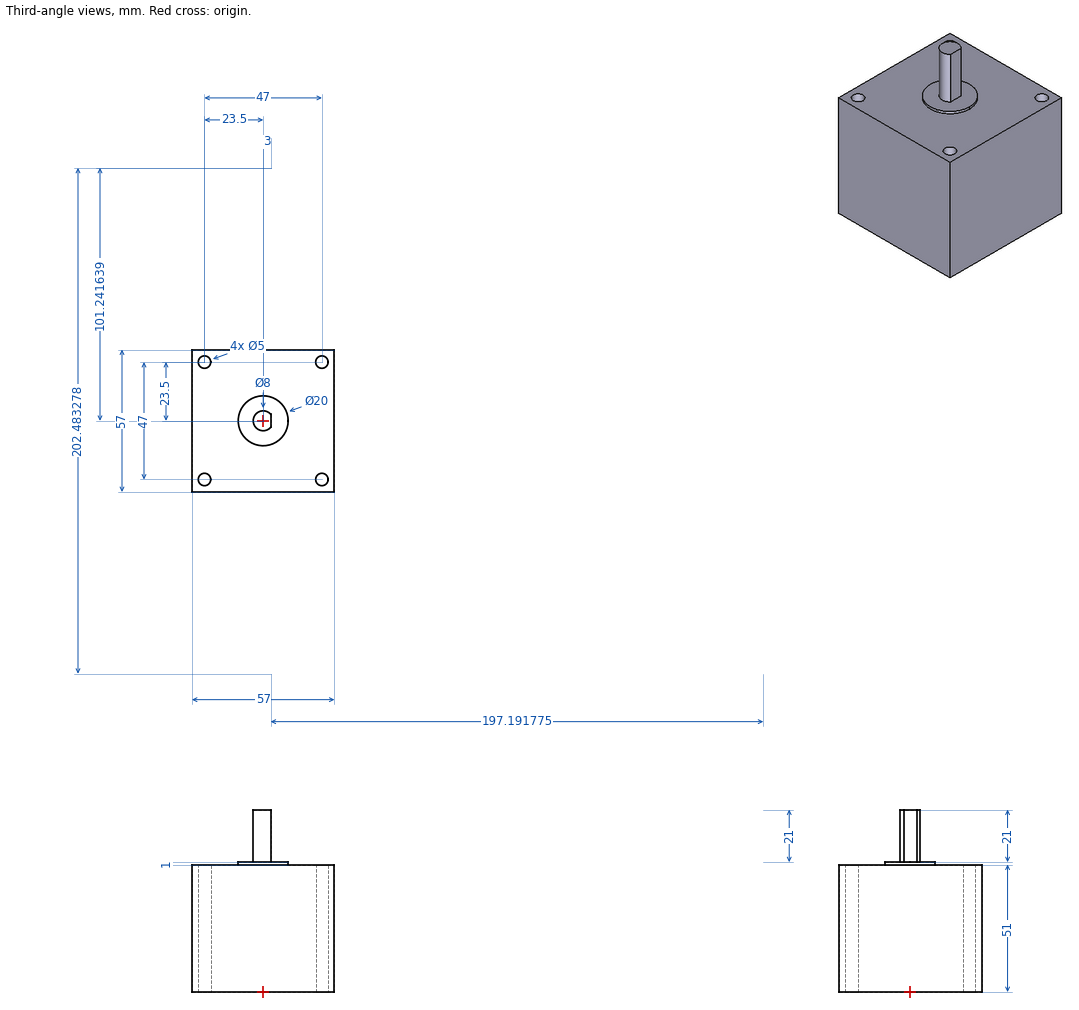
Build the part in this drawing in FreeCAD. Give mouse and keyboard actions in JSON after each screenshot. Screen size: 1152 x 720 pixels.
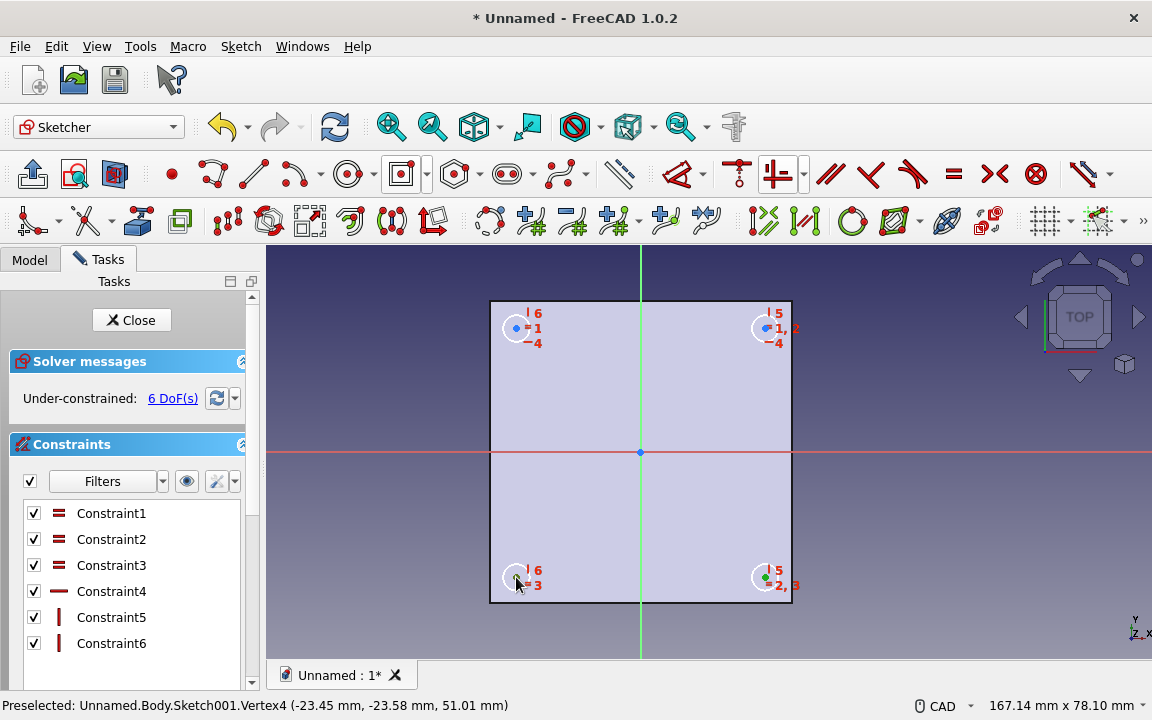
{"action": "left_click", "coordinate": [804, 174]}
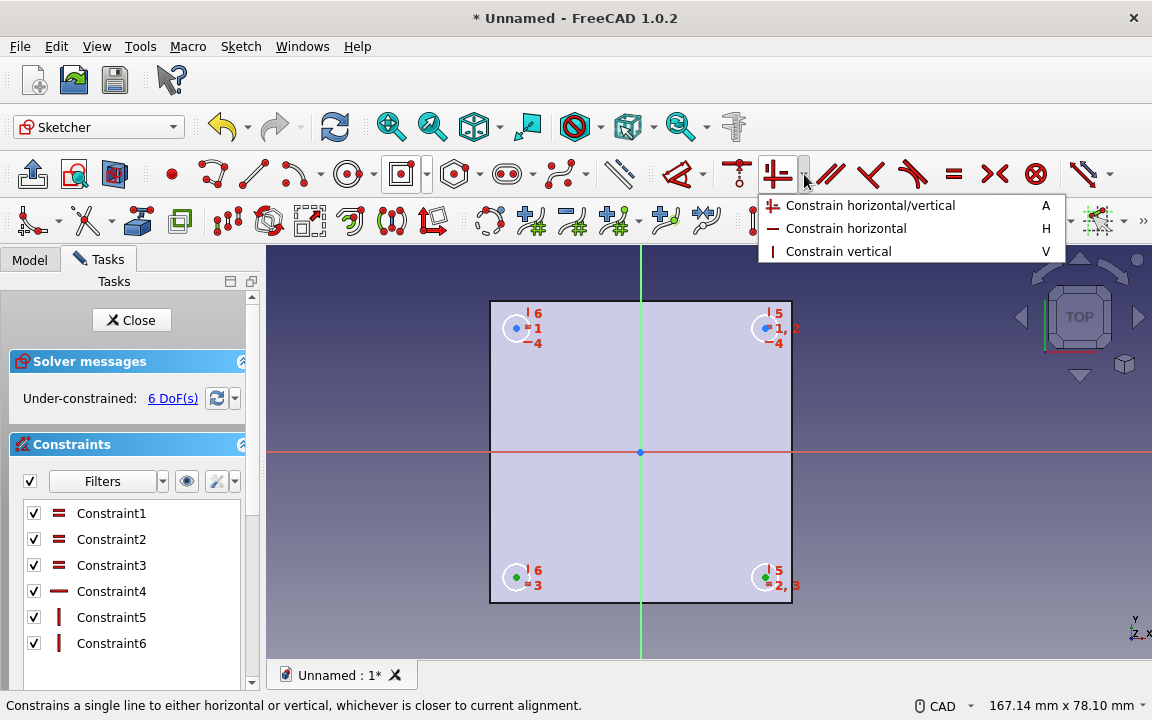
{"action": "left_click", "coordinate": [912, 228]}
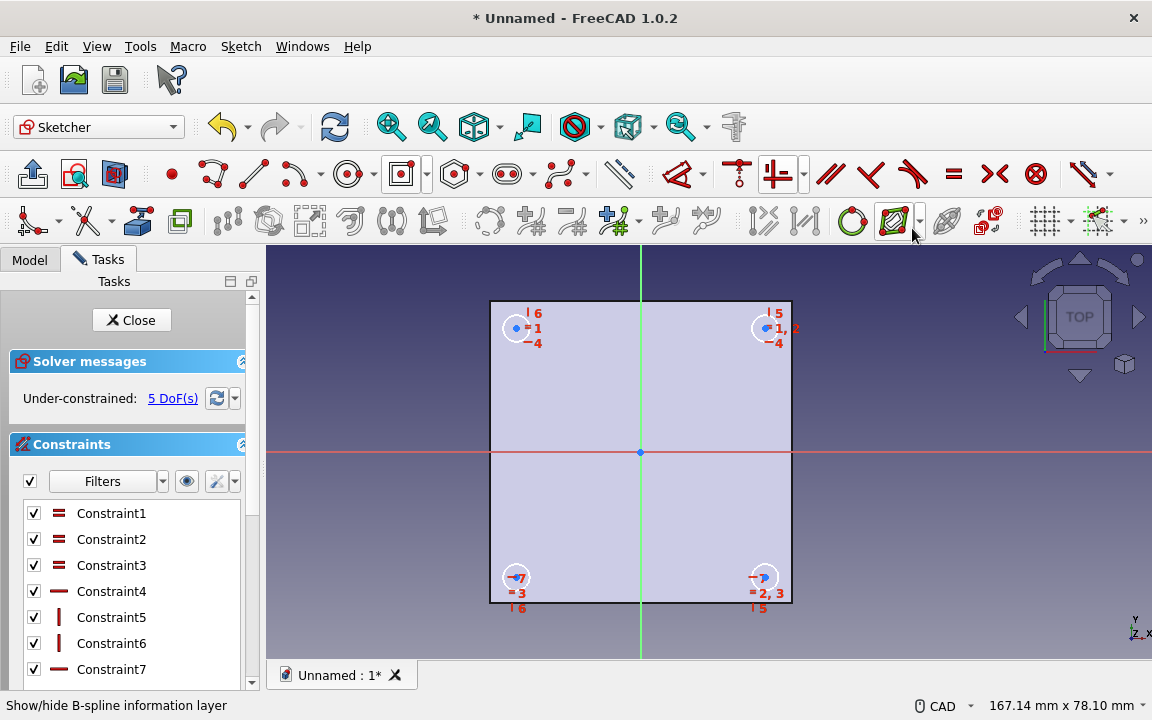
{"action": "left_click", "coordinate": [676, 174]}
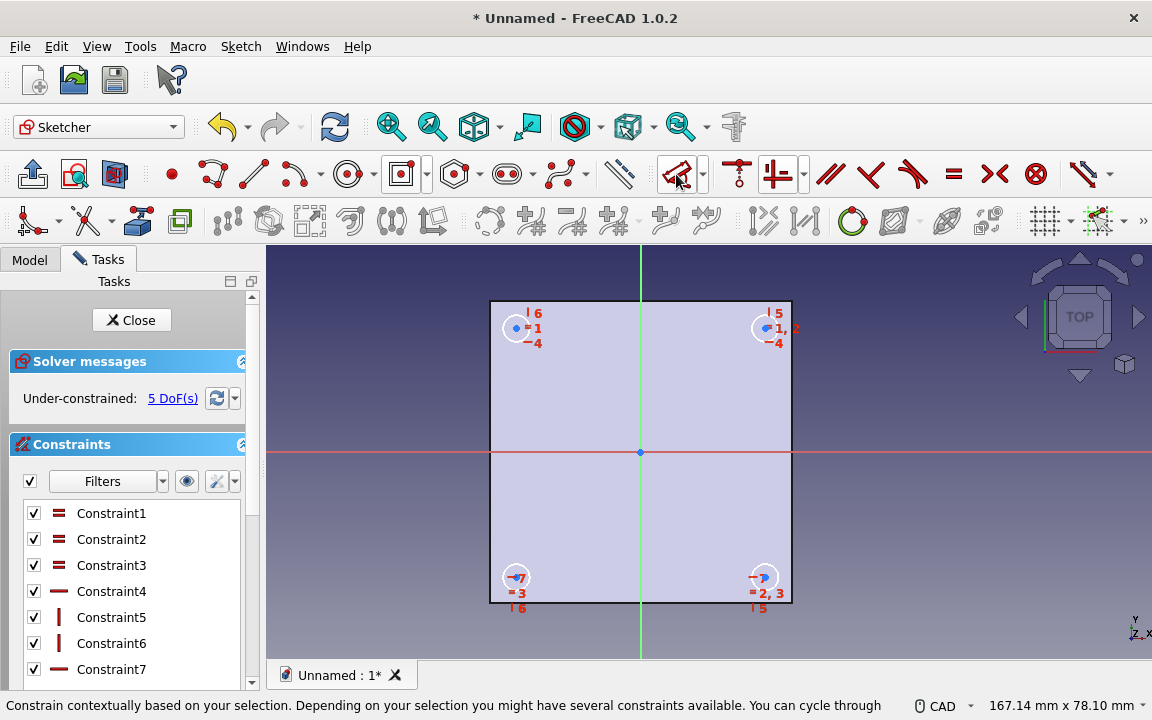
{"action": "scroll", "coordinate": [526, 319], "scroll_direction": "up", "scroll_amount": 3}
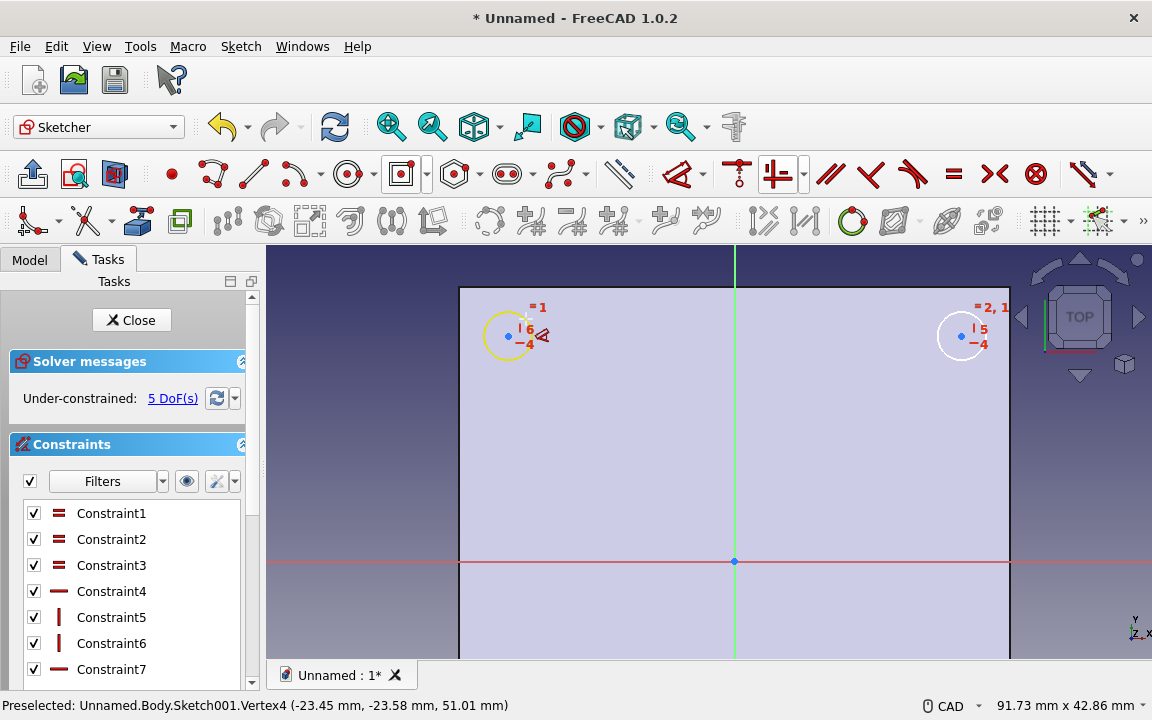
{"action": "left_click", "coordinate": [525, 319]}
{"action": "left_click", "coordinate": [547, 296]}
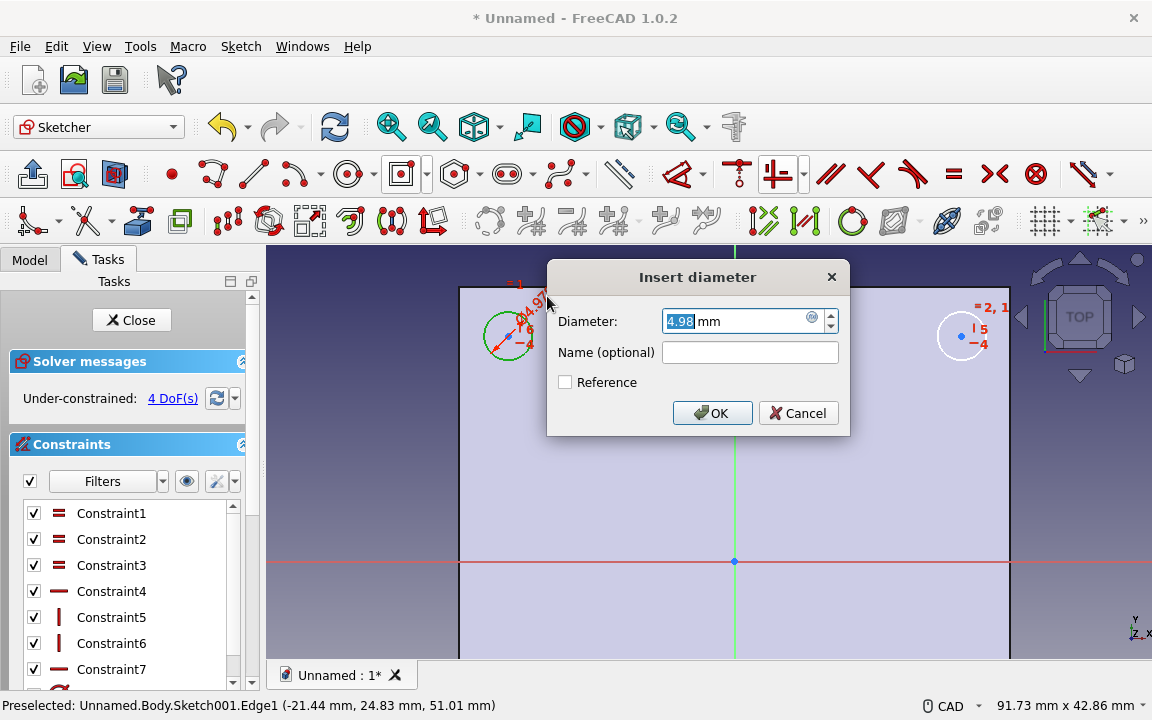
{"action": "type", "text": "5"}
{"action": "key", "text": "Return"}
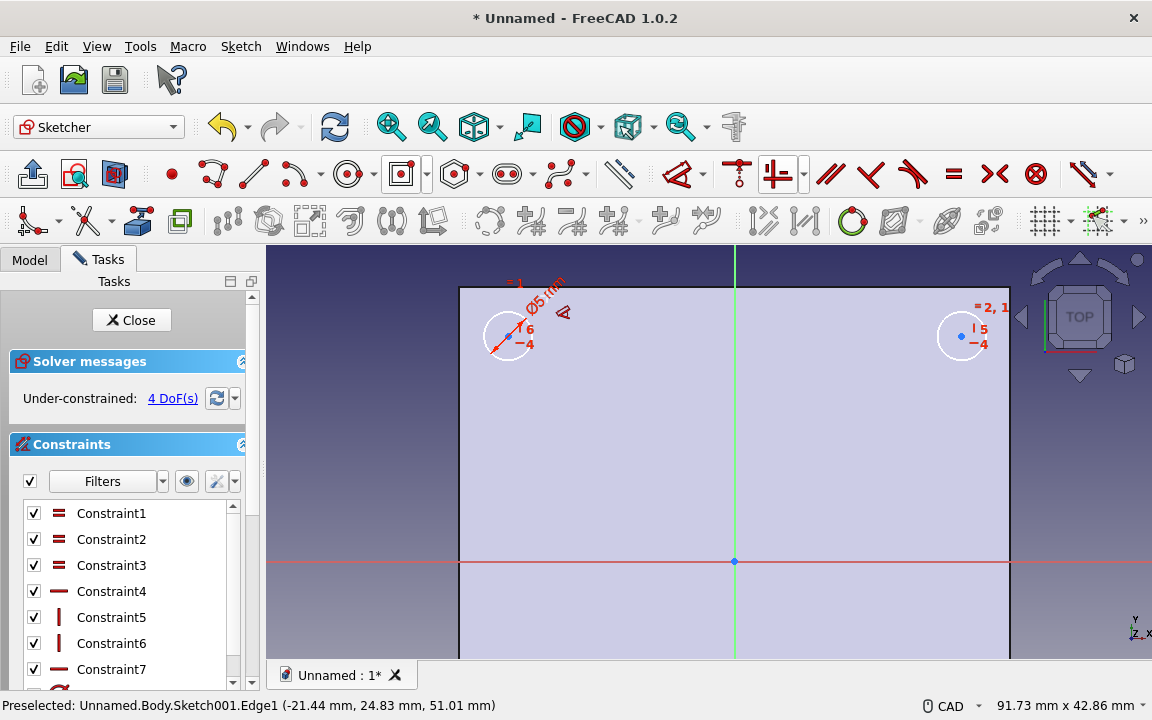
{"action": "left_click", "coordinate": [508, 336]}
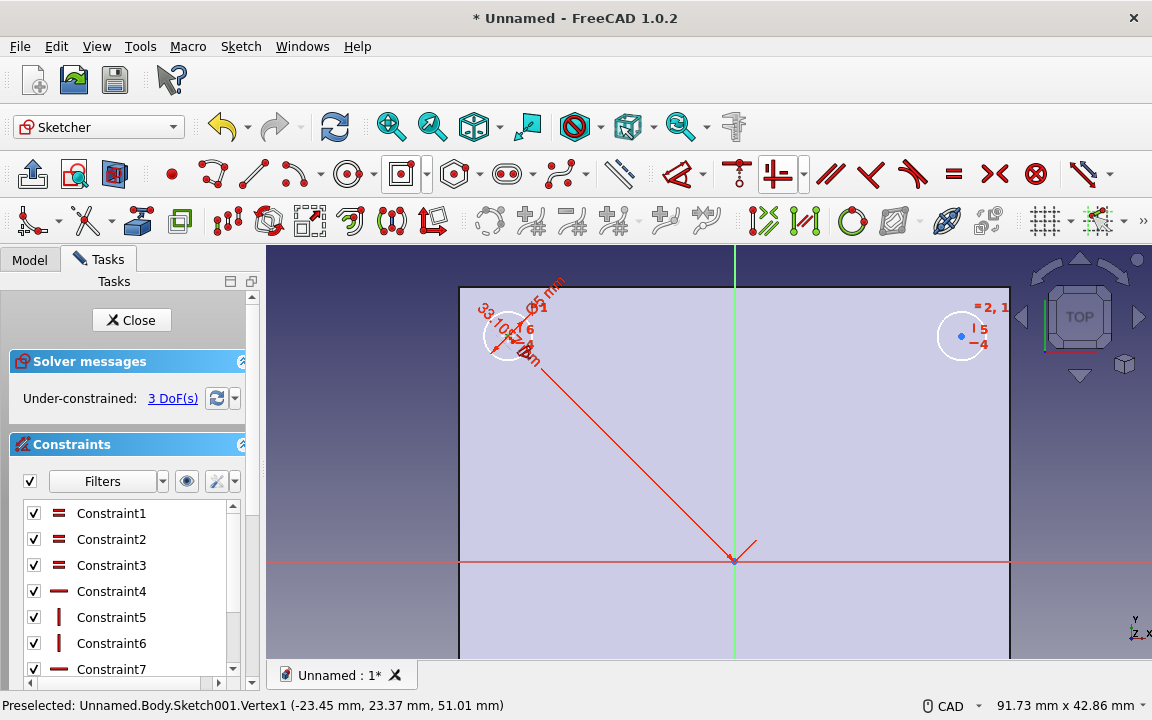
{"action": "left_click", "coordinate": [962, 336]}
{"action": "left_click", "coordinate": [631, 302]}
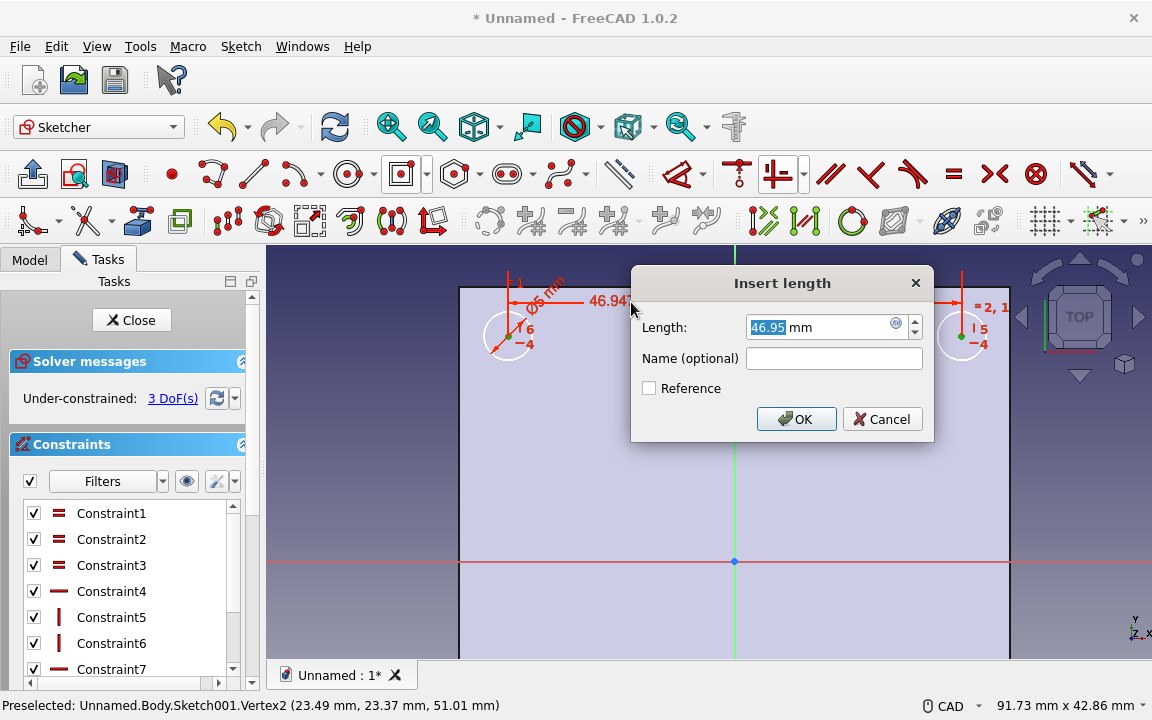
{"action": "type", "text": "47"}
{"action": "key", "text": "Return"}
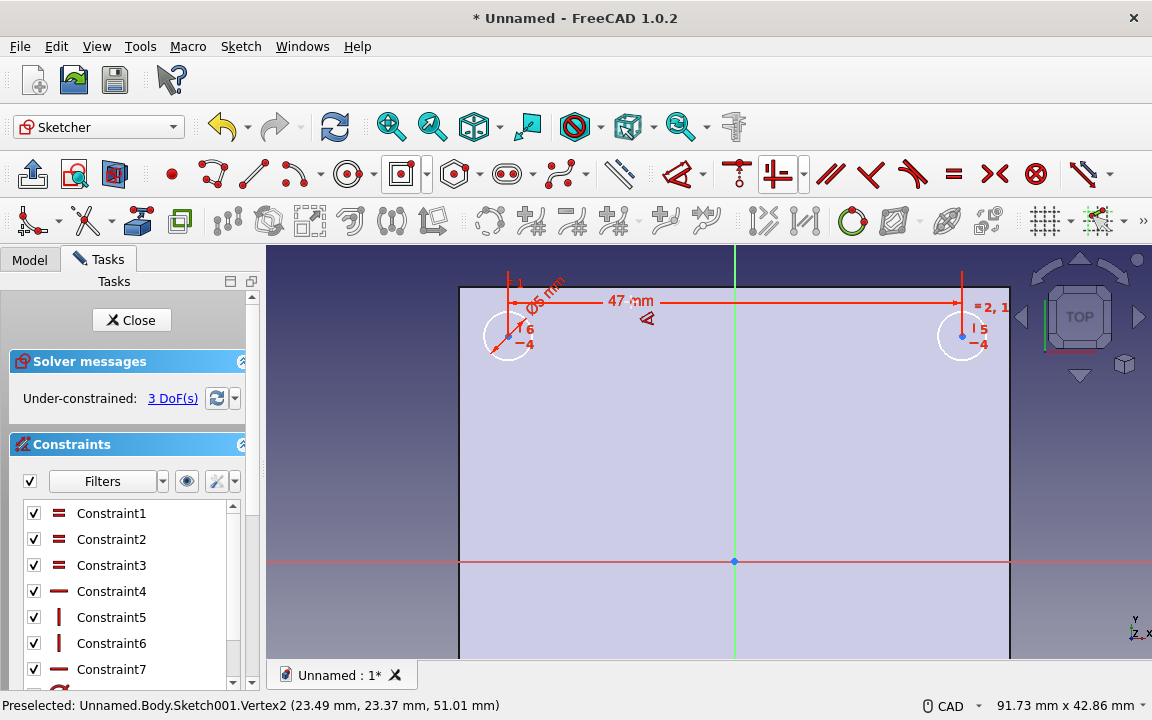
{"action": "left_click", "coordinate": [962, 336]}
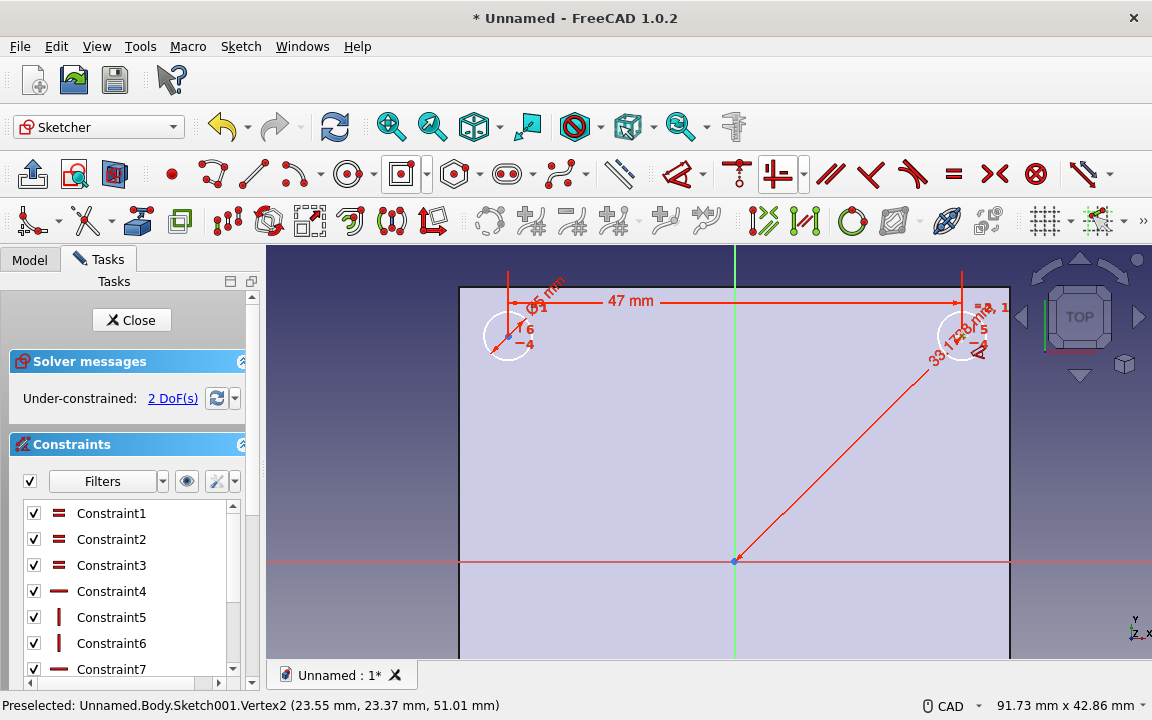
{"action": "scroll", "coordinate": [526, 318], "scroll_direction": "down", "scroll_amount": 3}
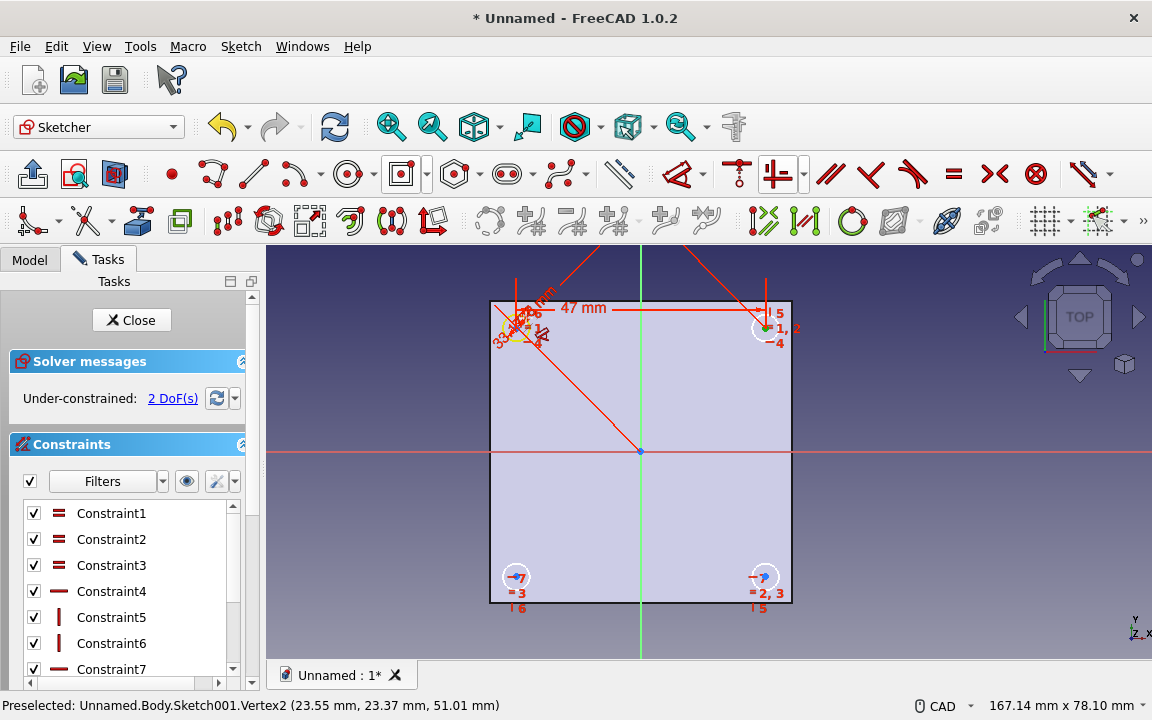
{"action": "left_click", "coordinate": [766, 577]}
{"action": "left_click", "coordinate": [800, 395]}